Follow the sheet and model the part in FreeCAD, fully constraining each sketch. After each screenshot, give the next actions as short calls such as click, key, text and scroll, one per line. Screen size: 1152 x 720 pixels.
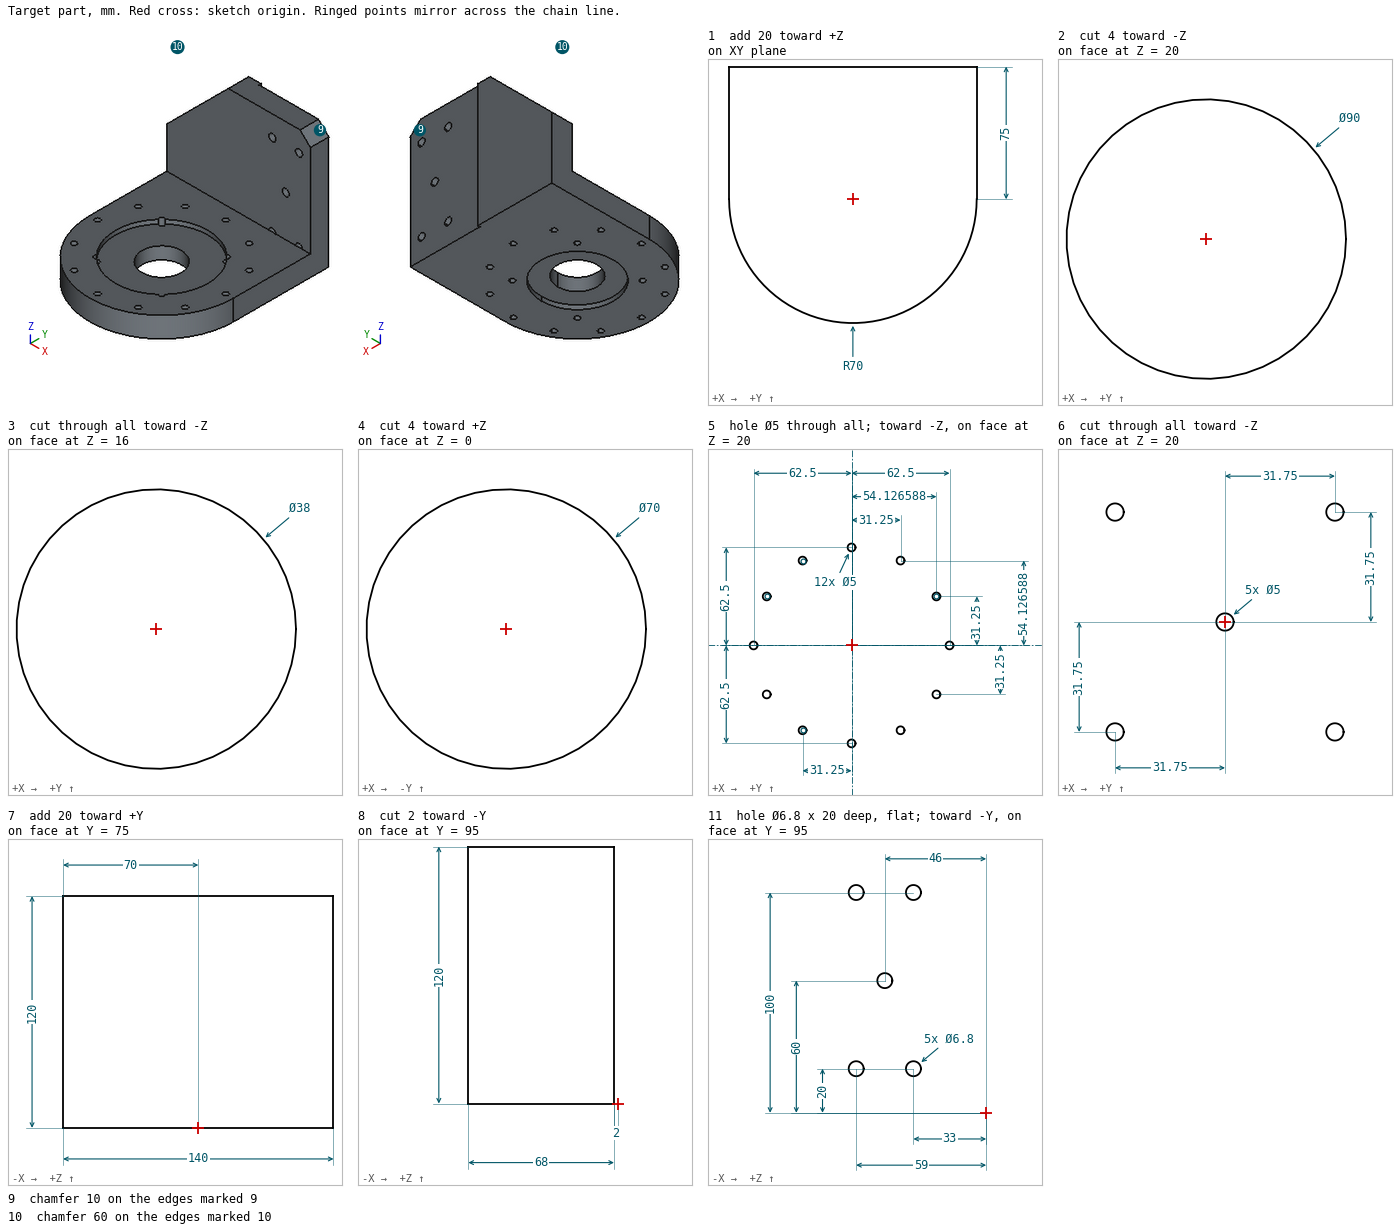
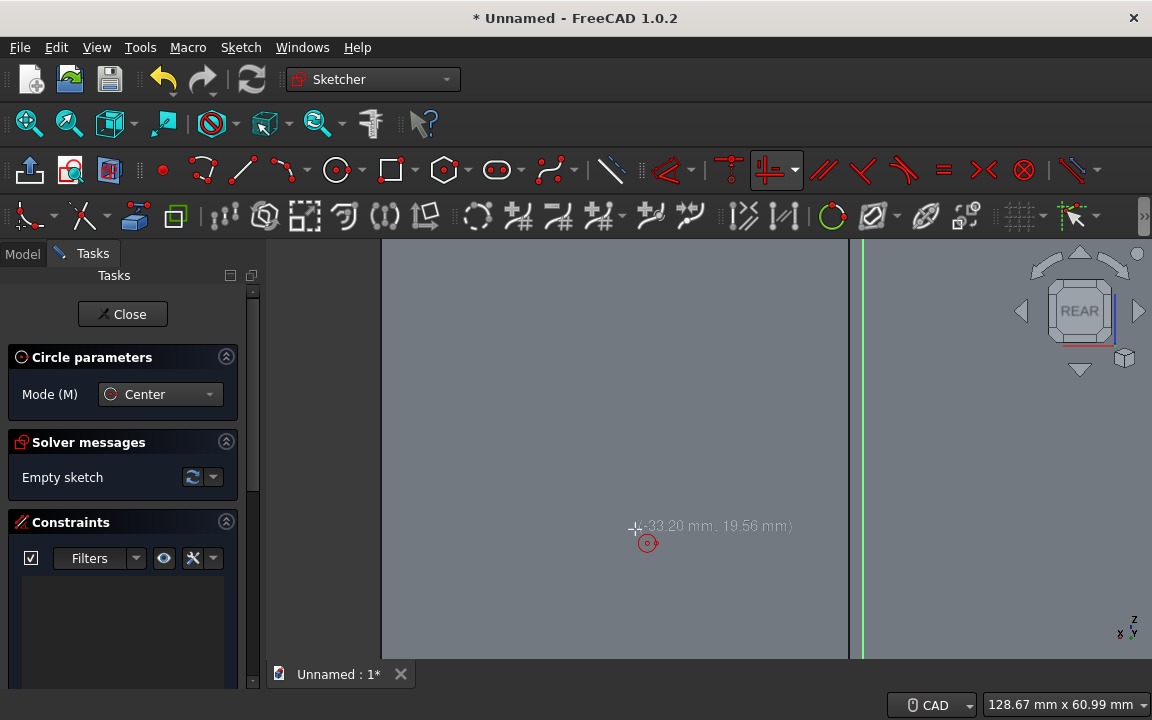
click(636, 527)
move(652, 511)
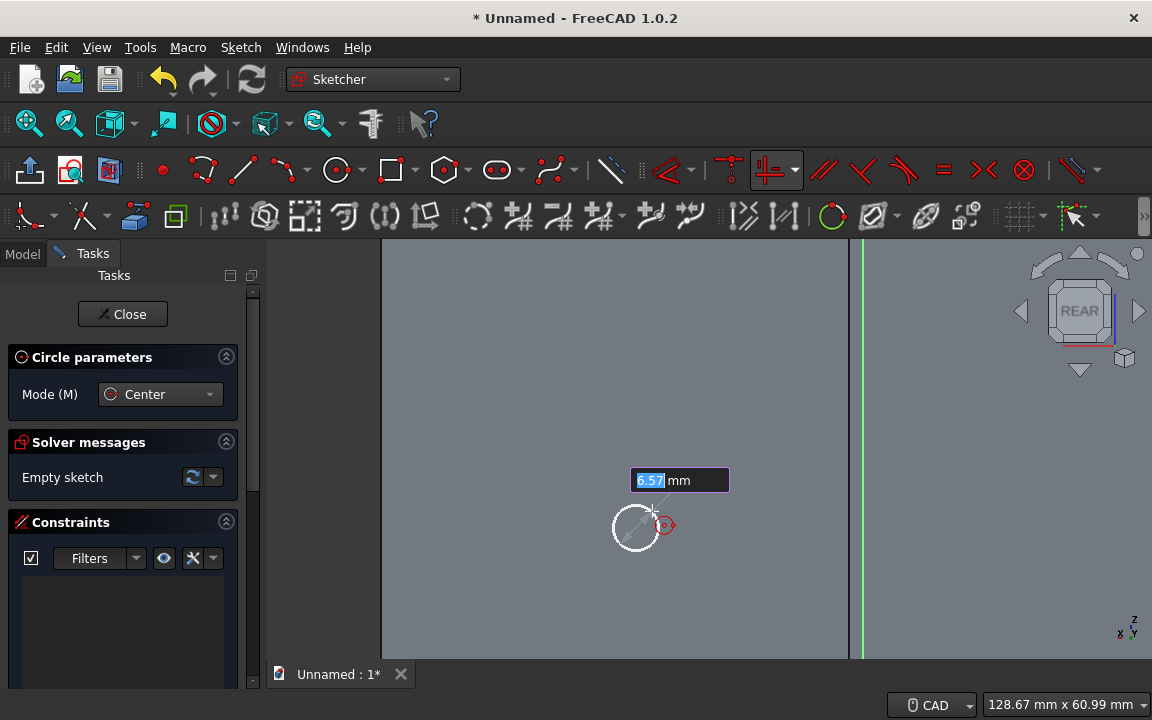
text(6.8)
key(Return)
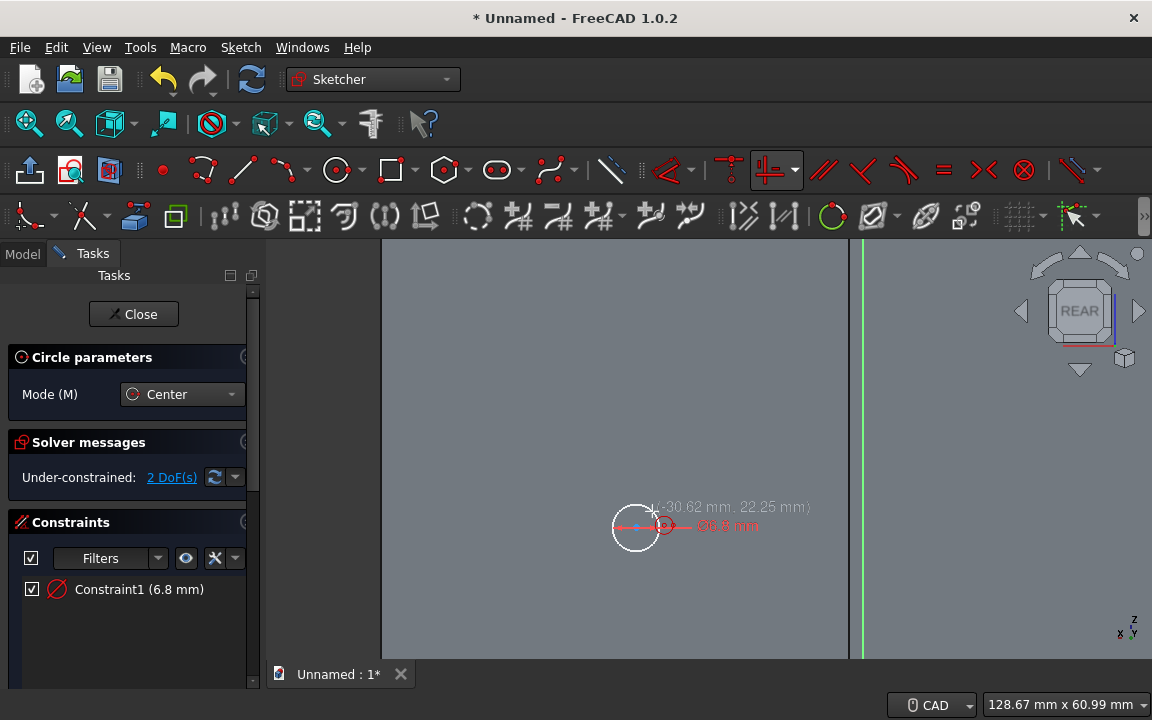
click(457, 527)
move(473, 511)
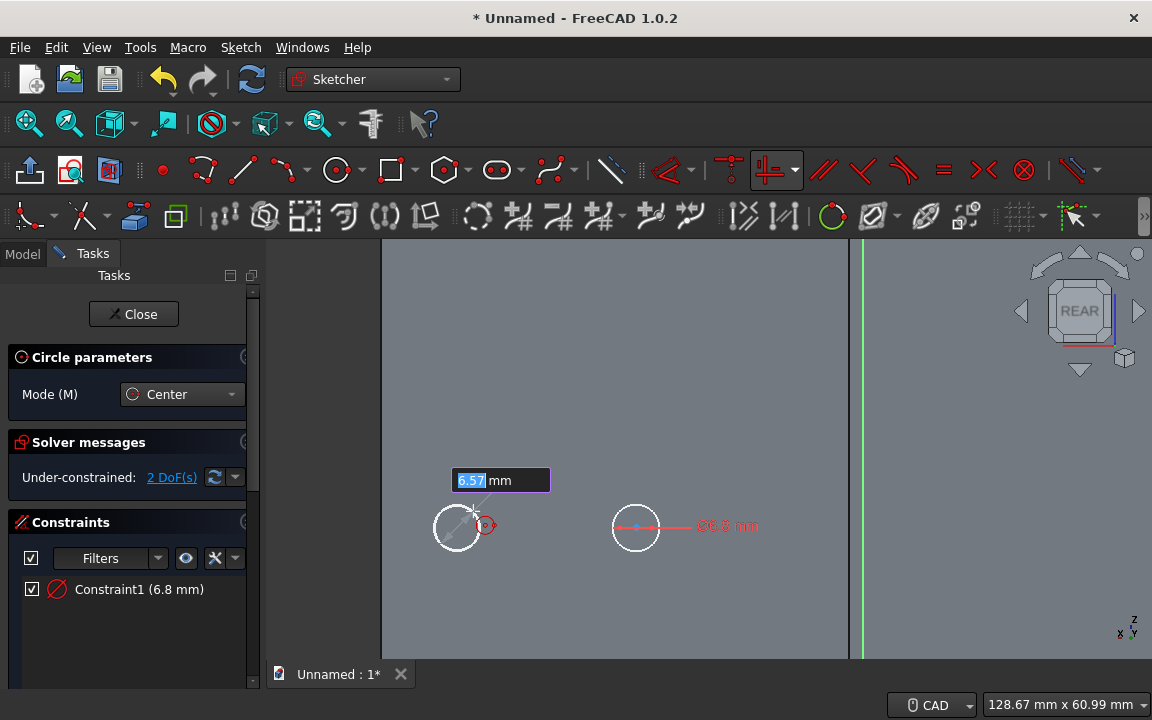
text(6.8)
key(Return)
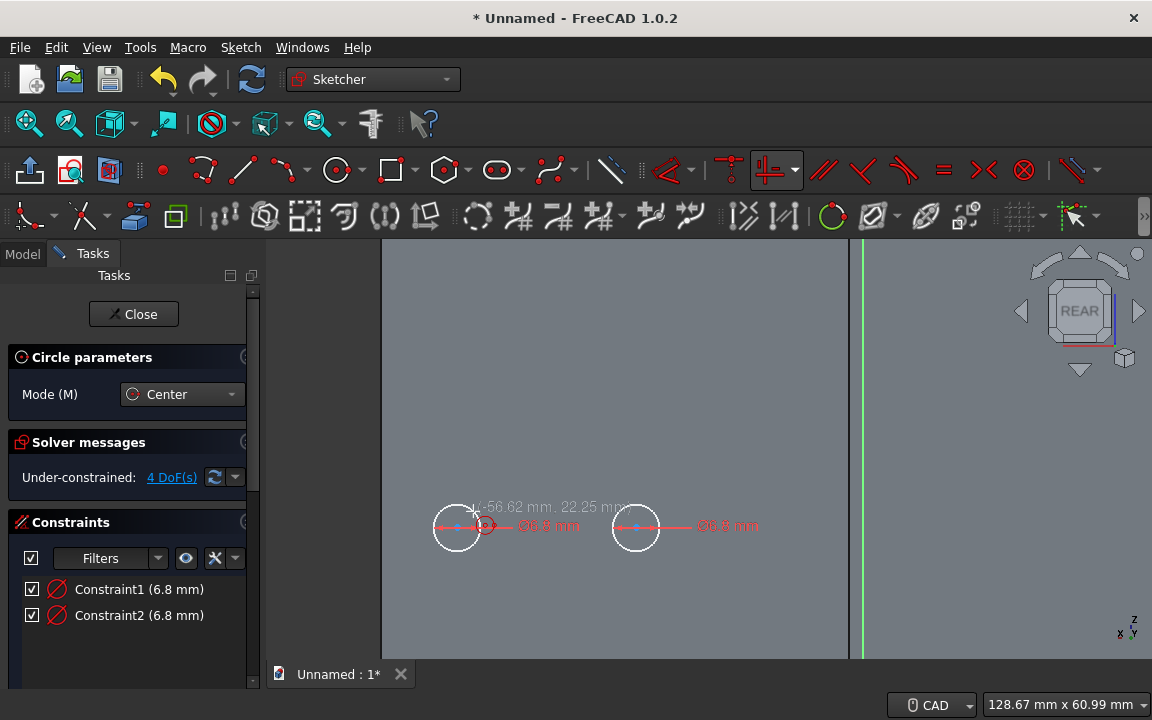
scroll(636, 530, down, 5)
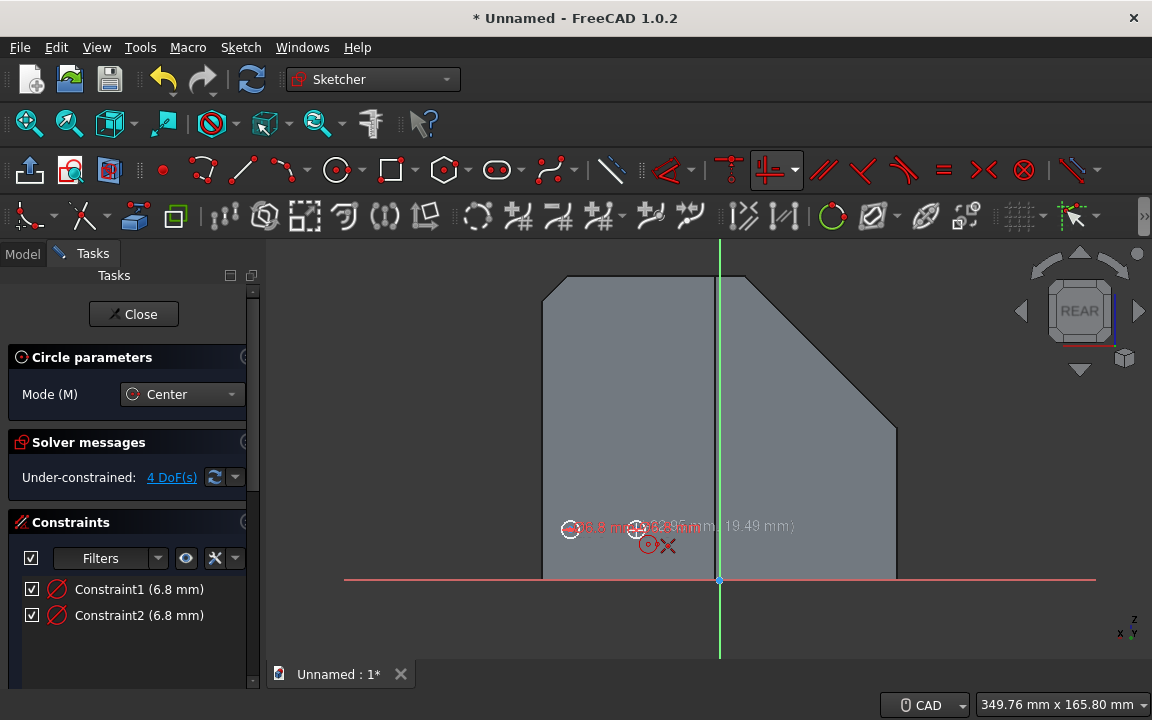
scroll(603, 428, up, 5)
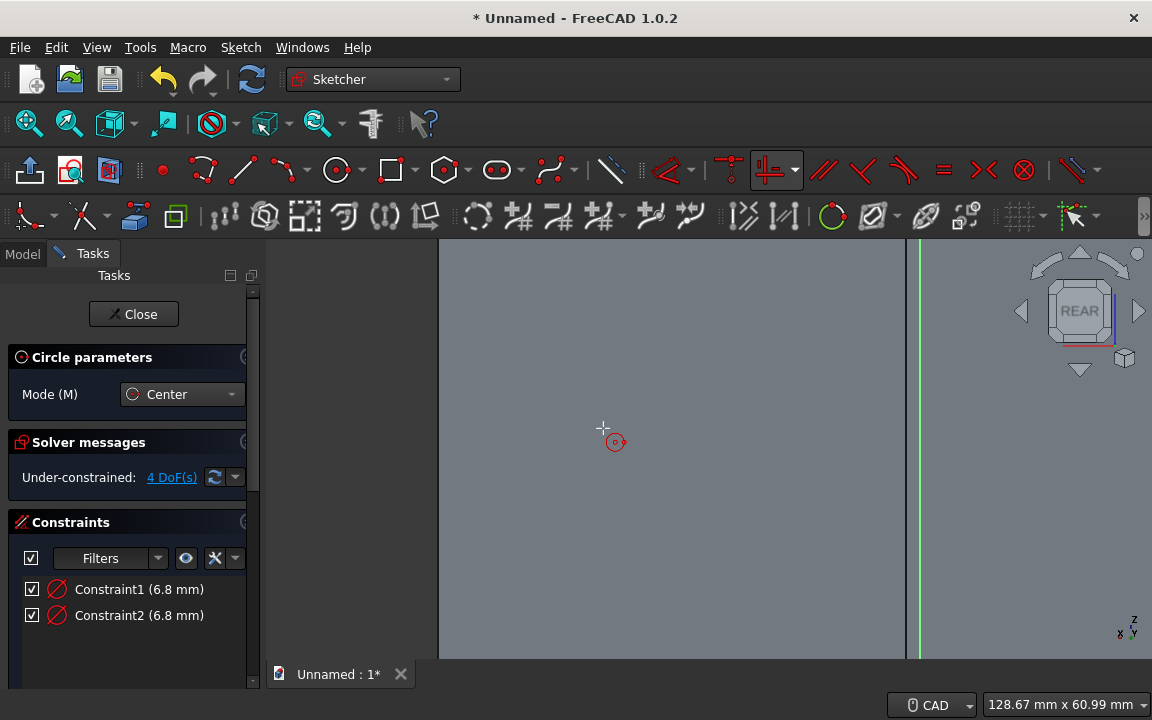
click(603, 428)
move(619, 411)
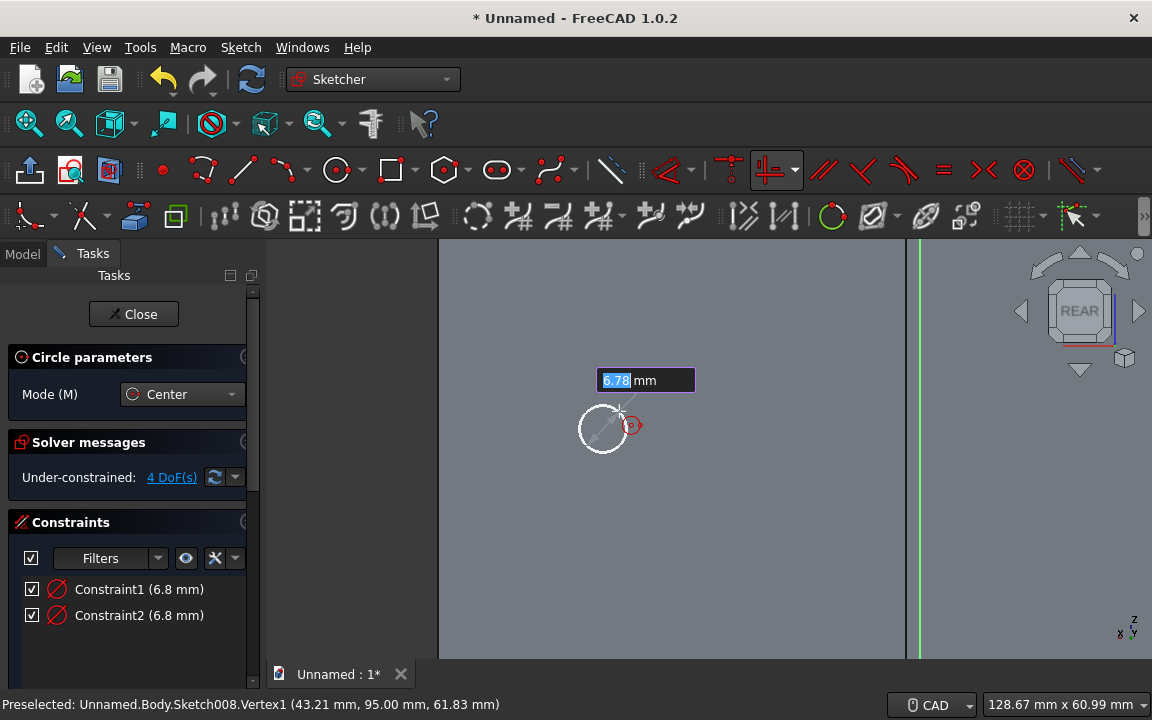
text(6.8)
key(Return)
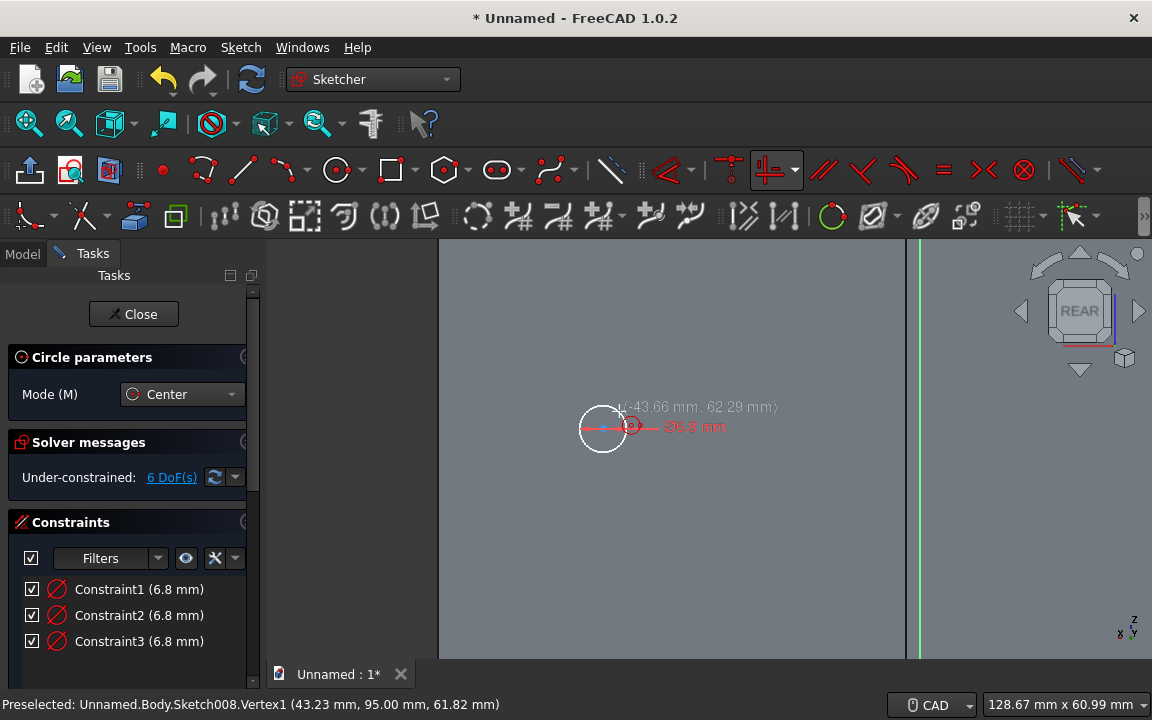
scroll(603, 428, down, 5)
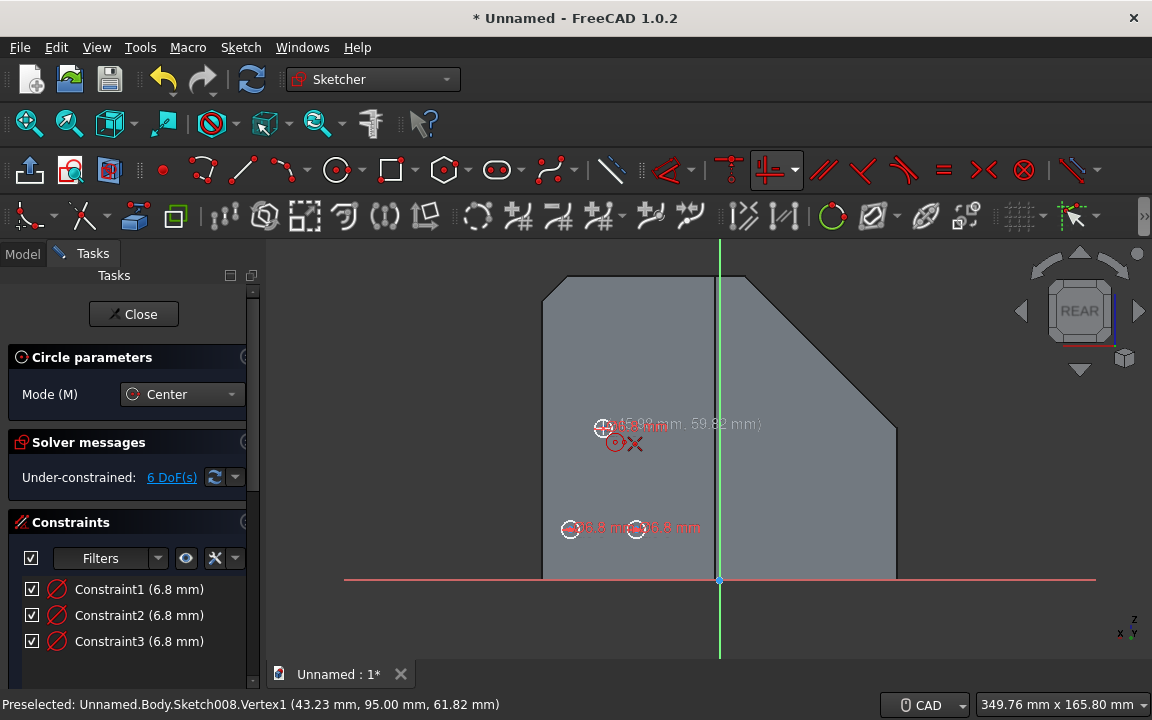
scroll(636, 327, up, 5)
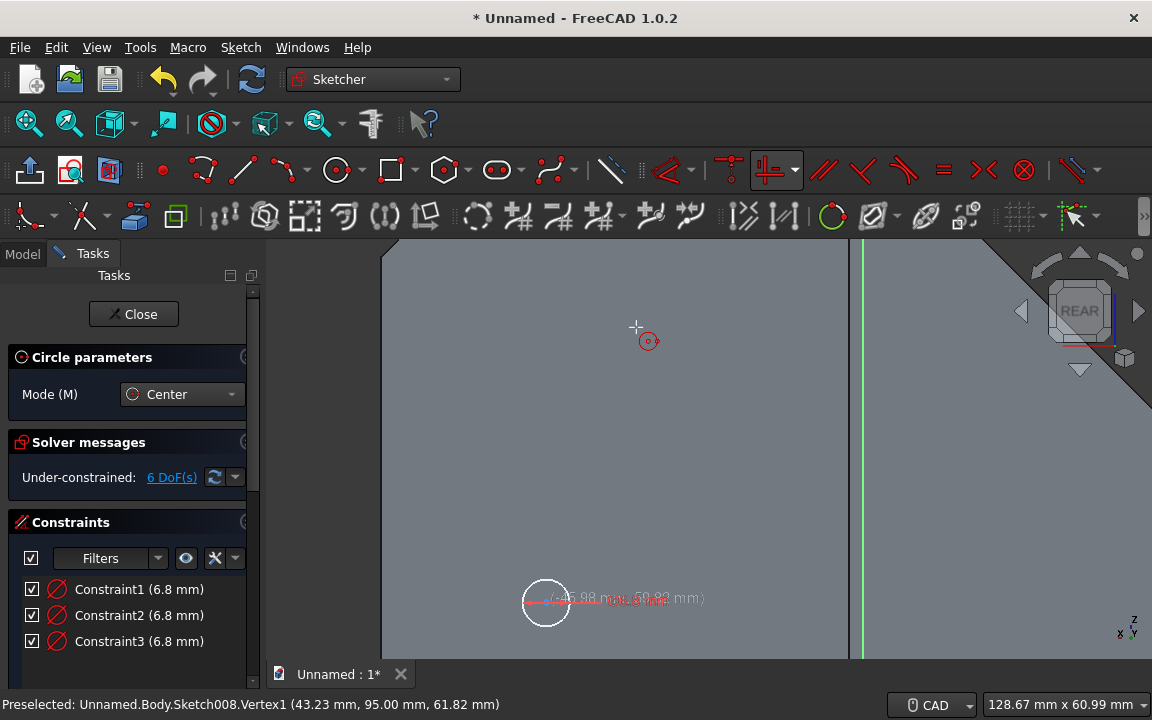
click(636, 326)
move(652, 310)